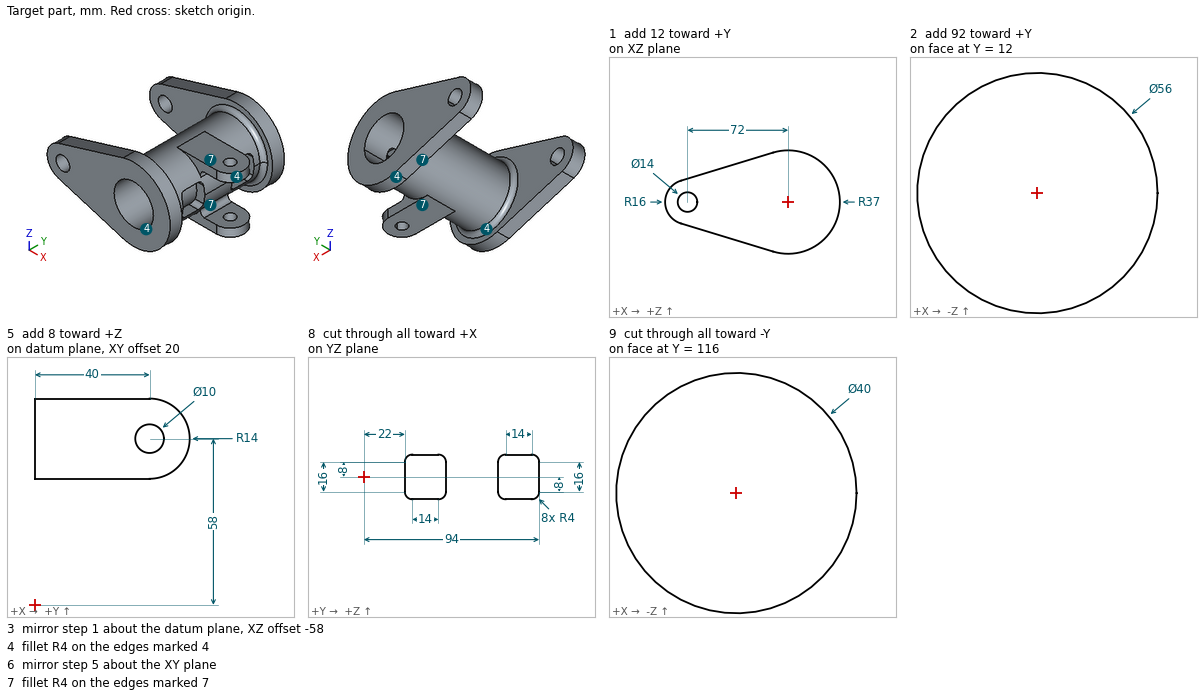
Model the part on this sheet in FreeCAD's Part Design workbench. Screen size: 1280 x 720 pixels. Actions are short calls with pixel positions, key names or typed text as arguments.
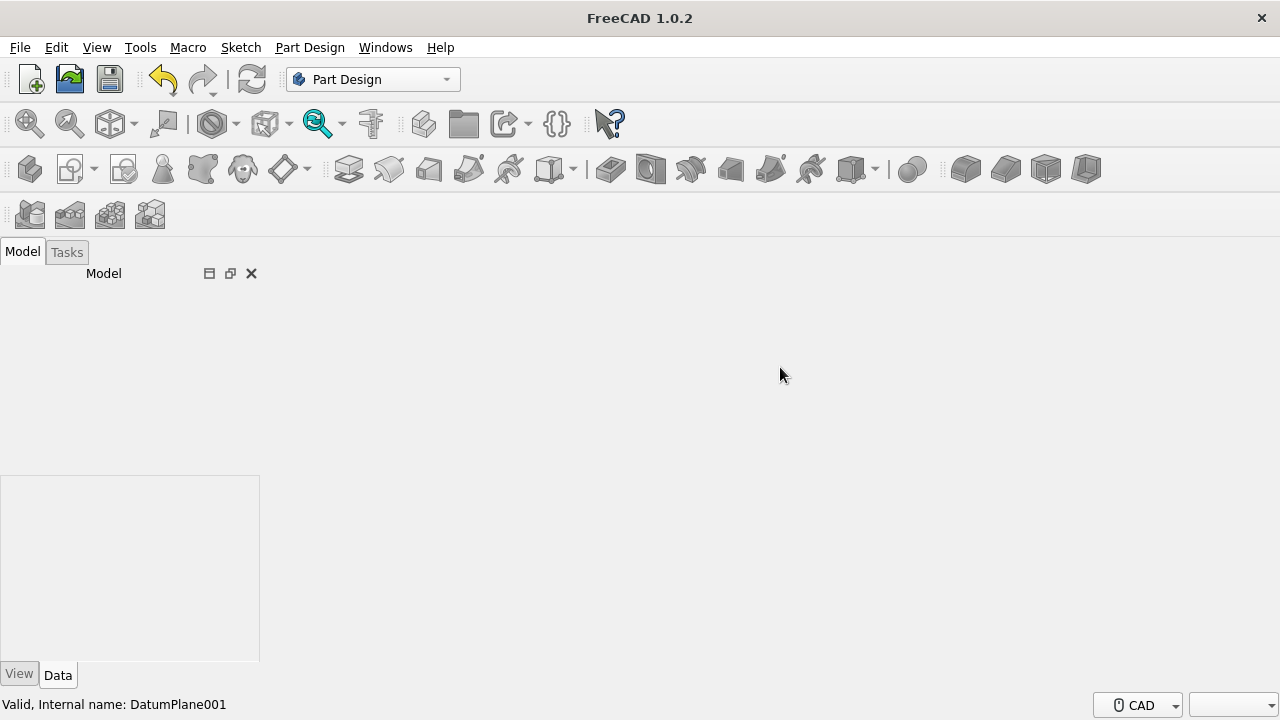
click(30, 80)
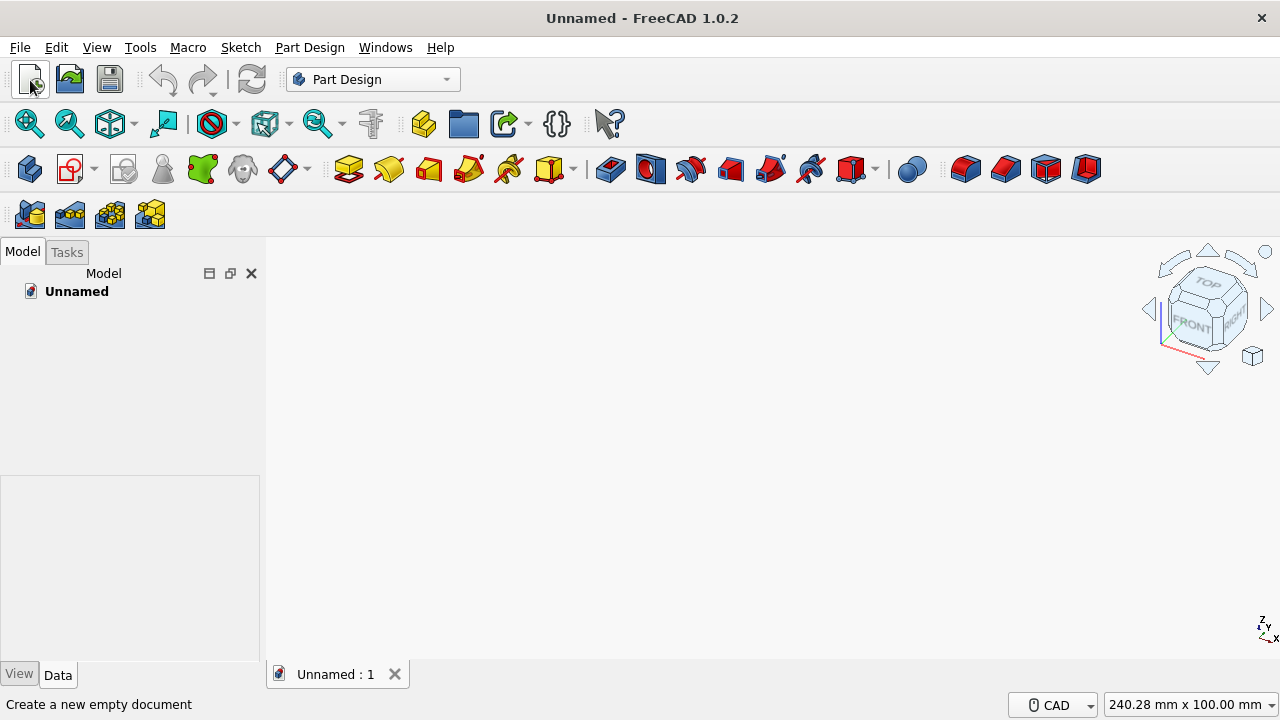
click(70, 170)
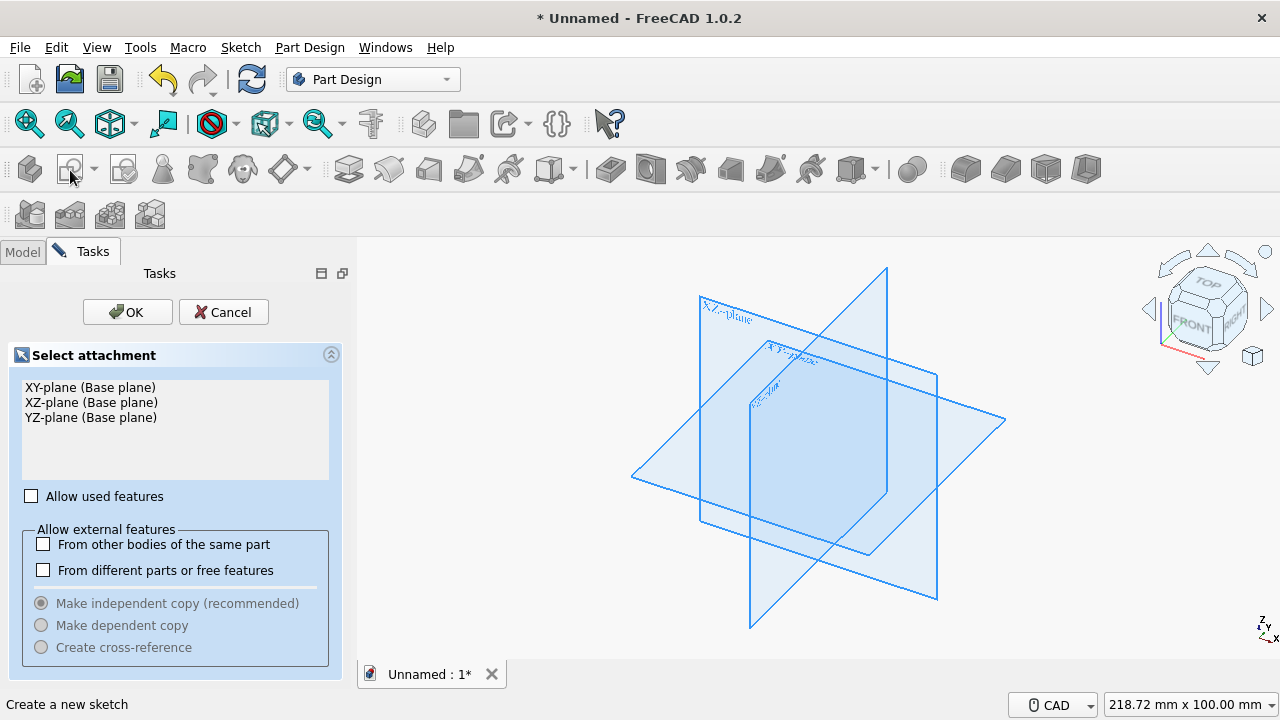
click(82, 402)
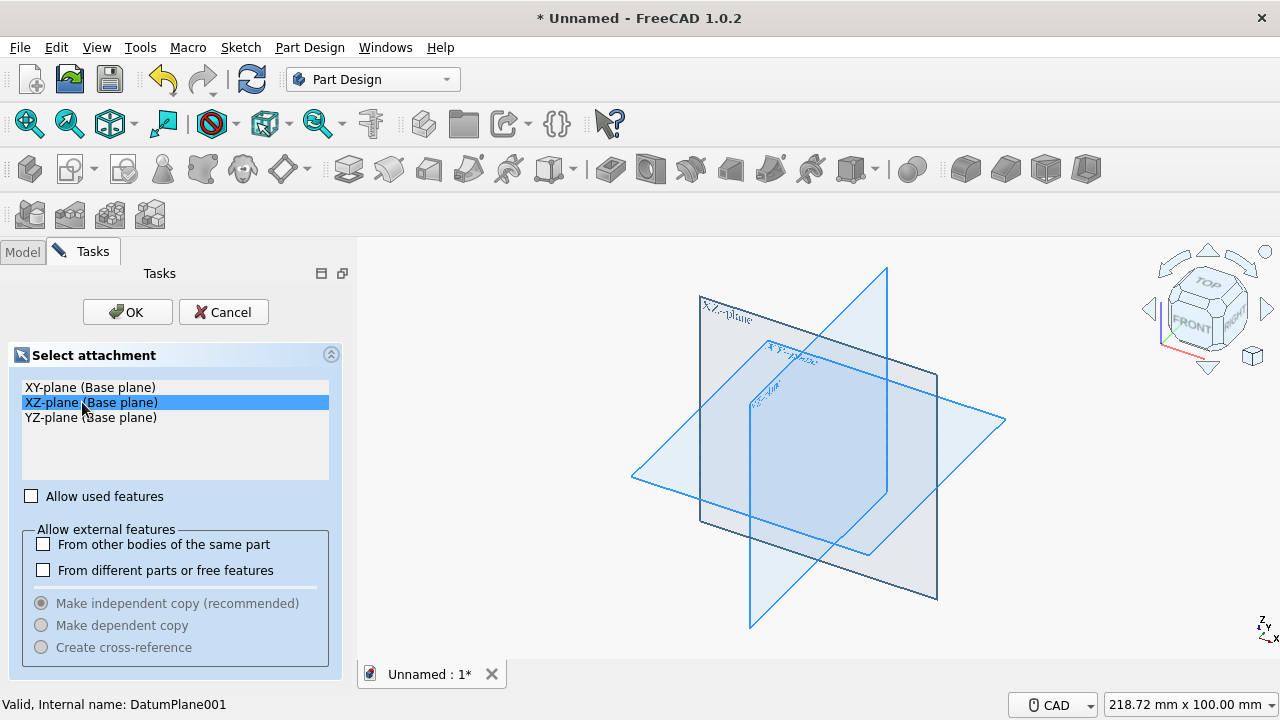
click(128, 312)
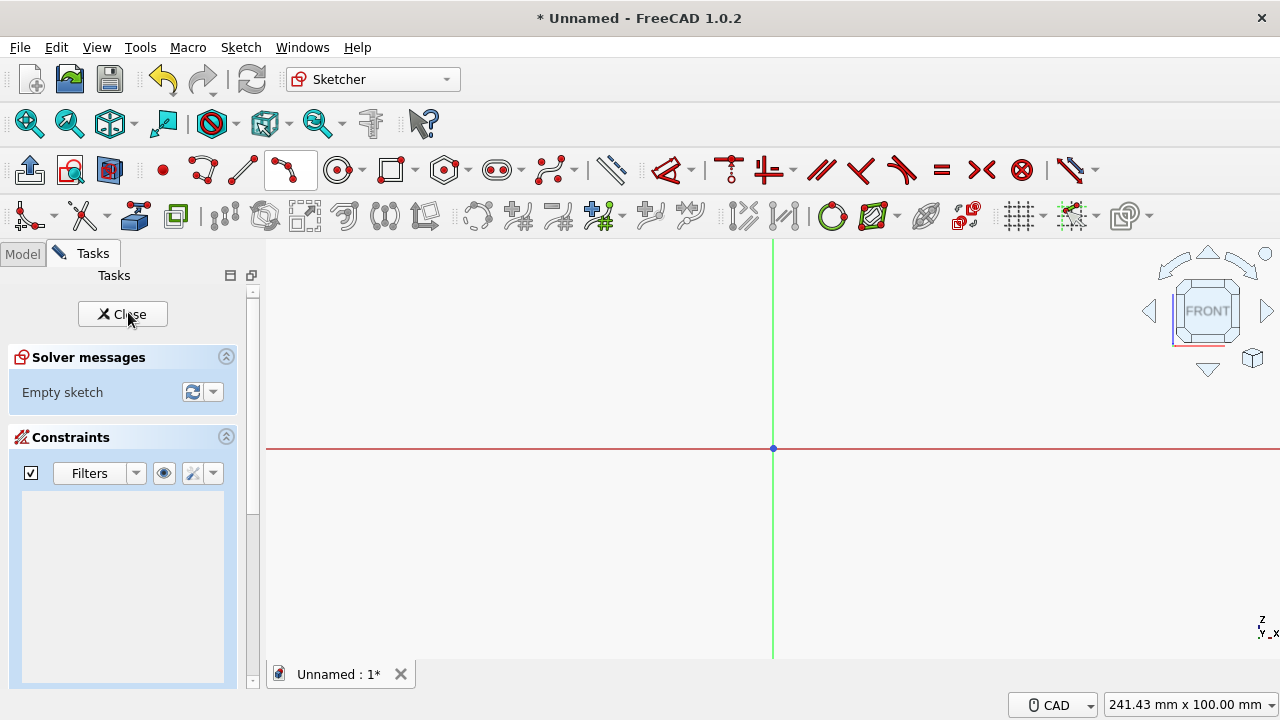
click(244, 170)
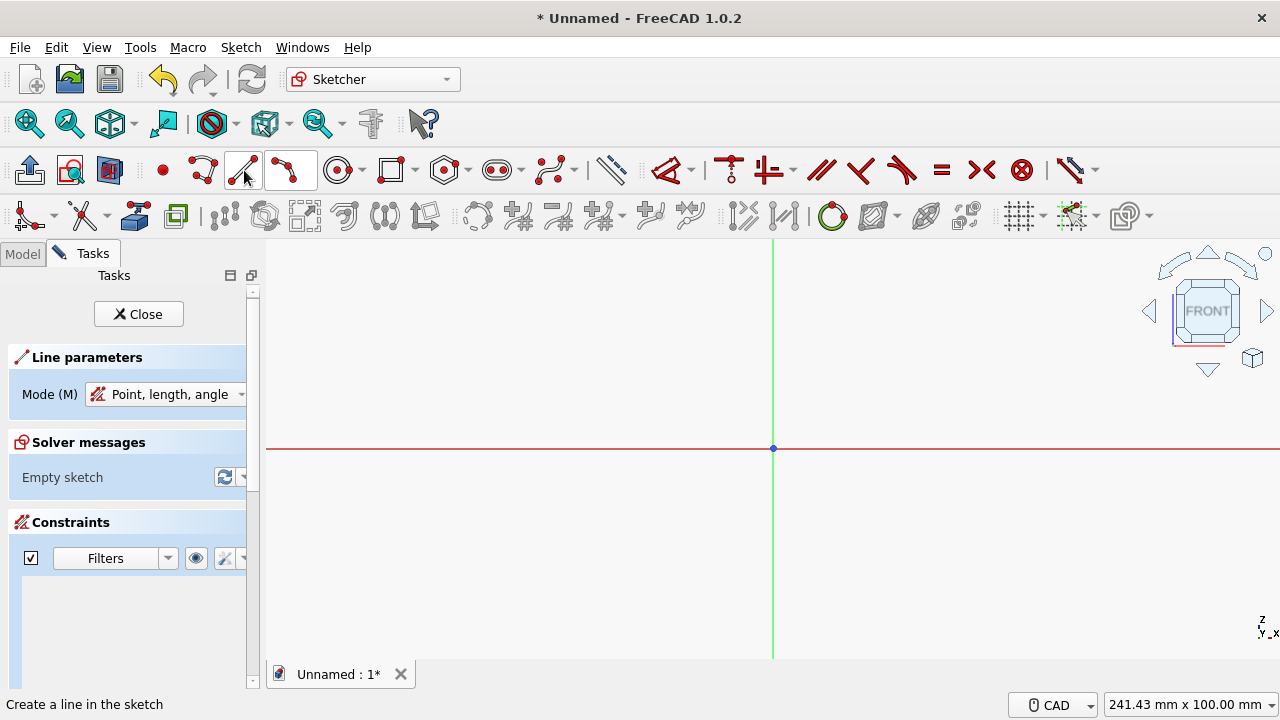
click(728, 598)
click(451, 513)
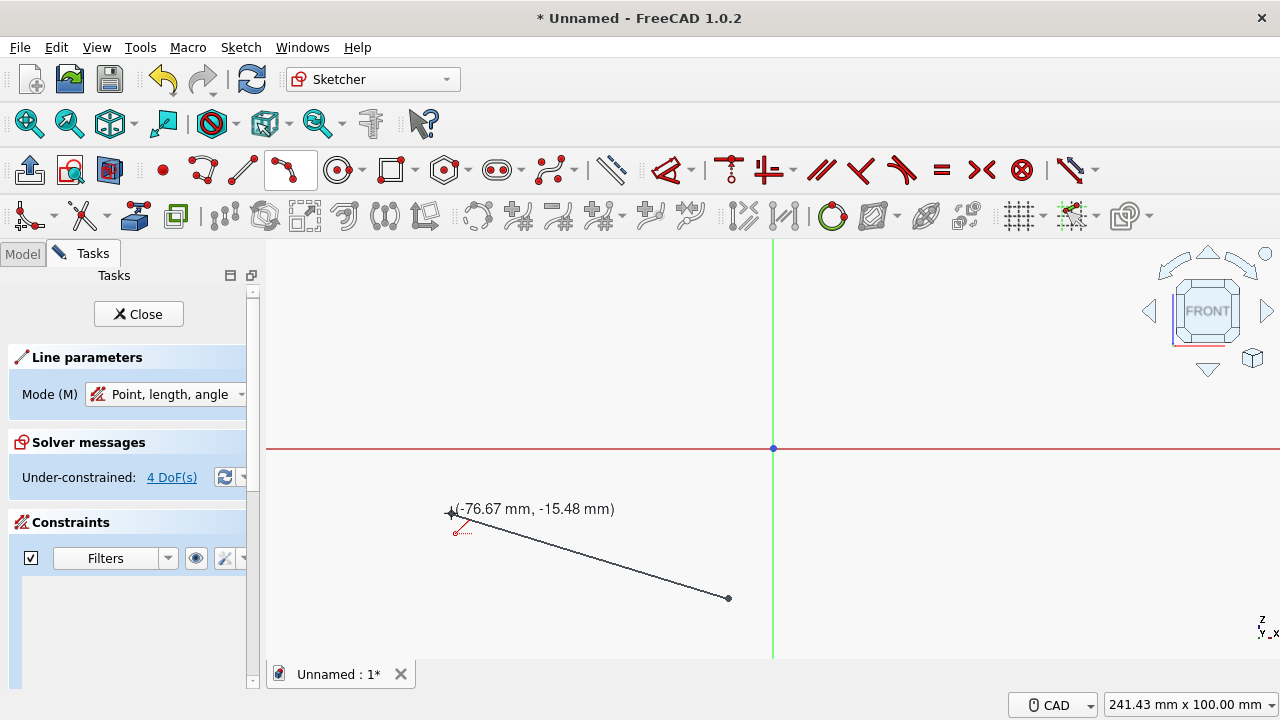
click(451, 385)
click(728, 300)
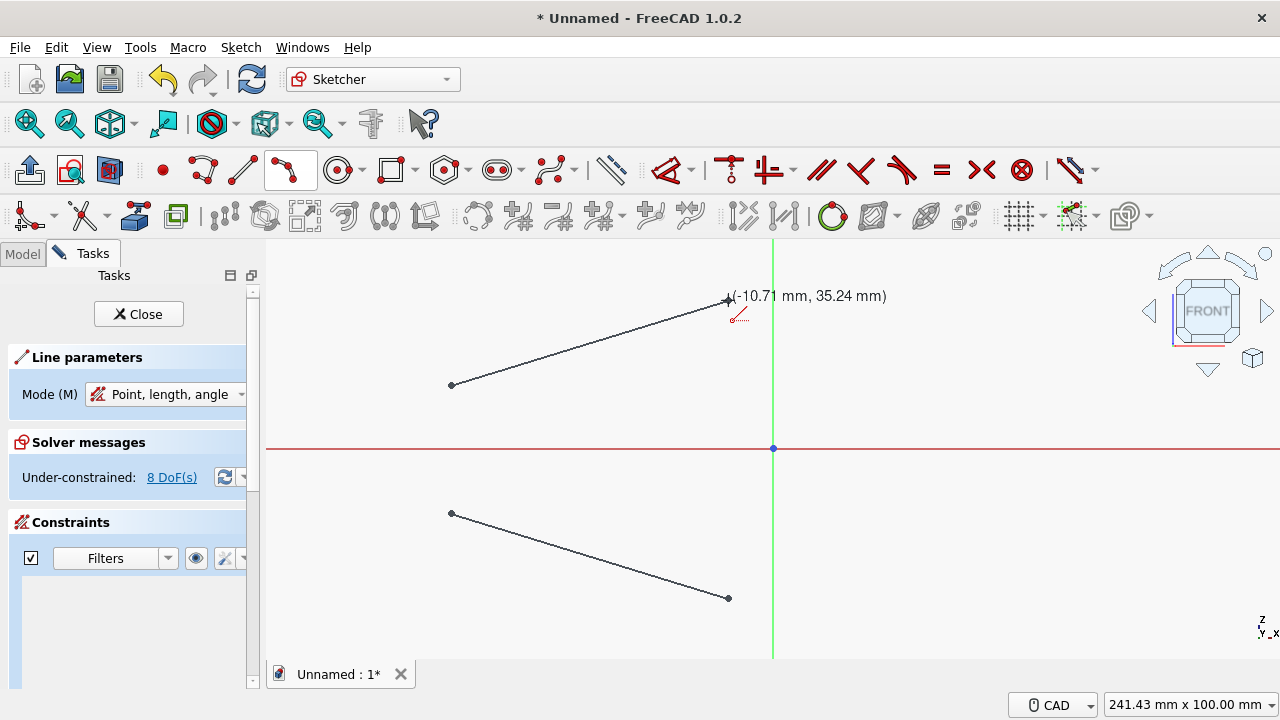
click(284, 170)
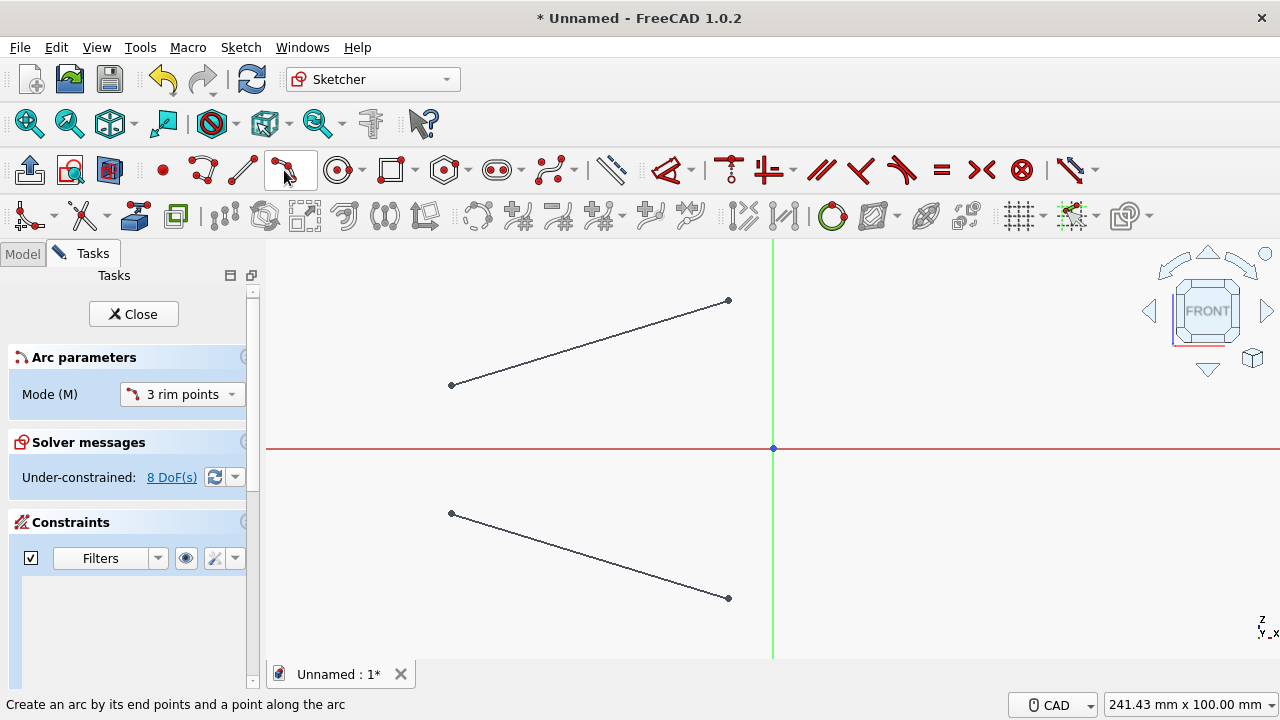
click(451, 514)
click(451, 386)
click(406, 432)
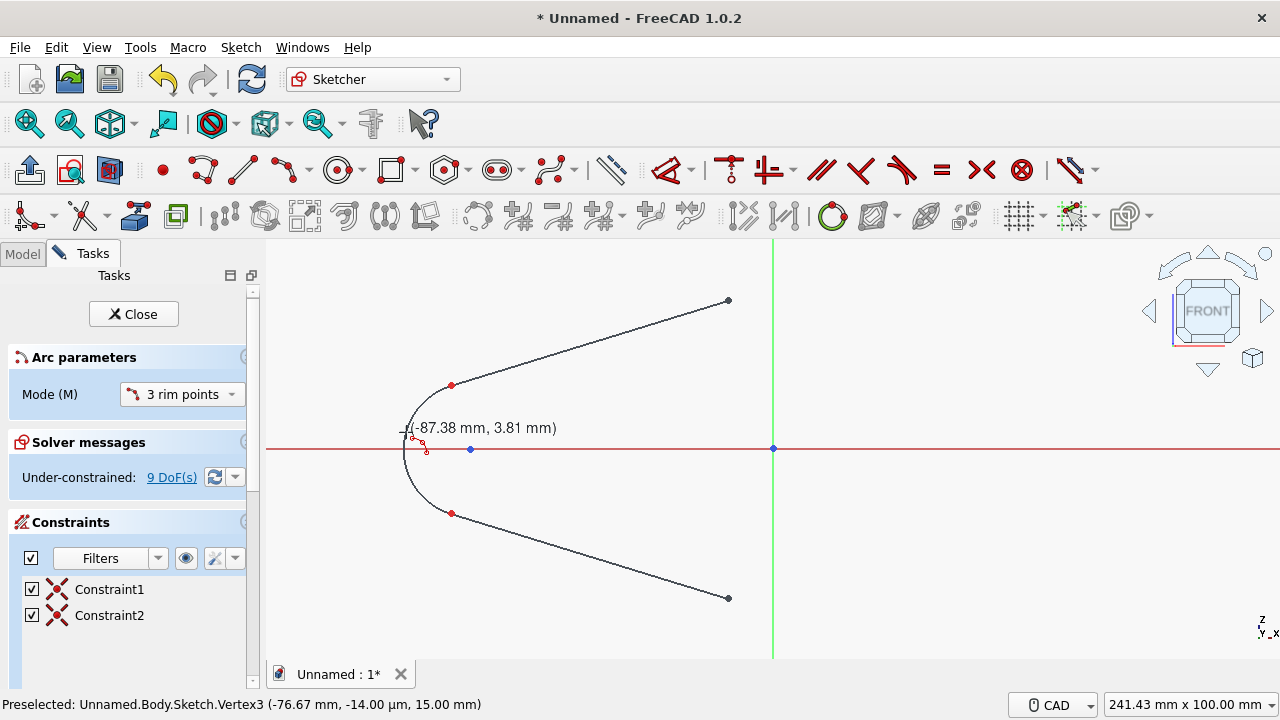
click(728, 301)
click(728, 599)
click(918, 506)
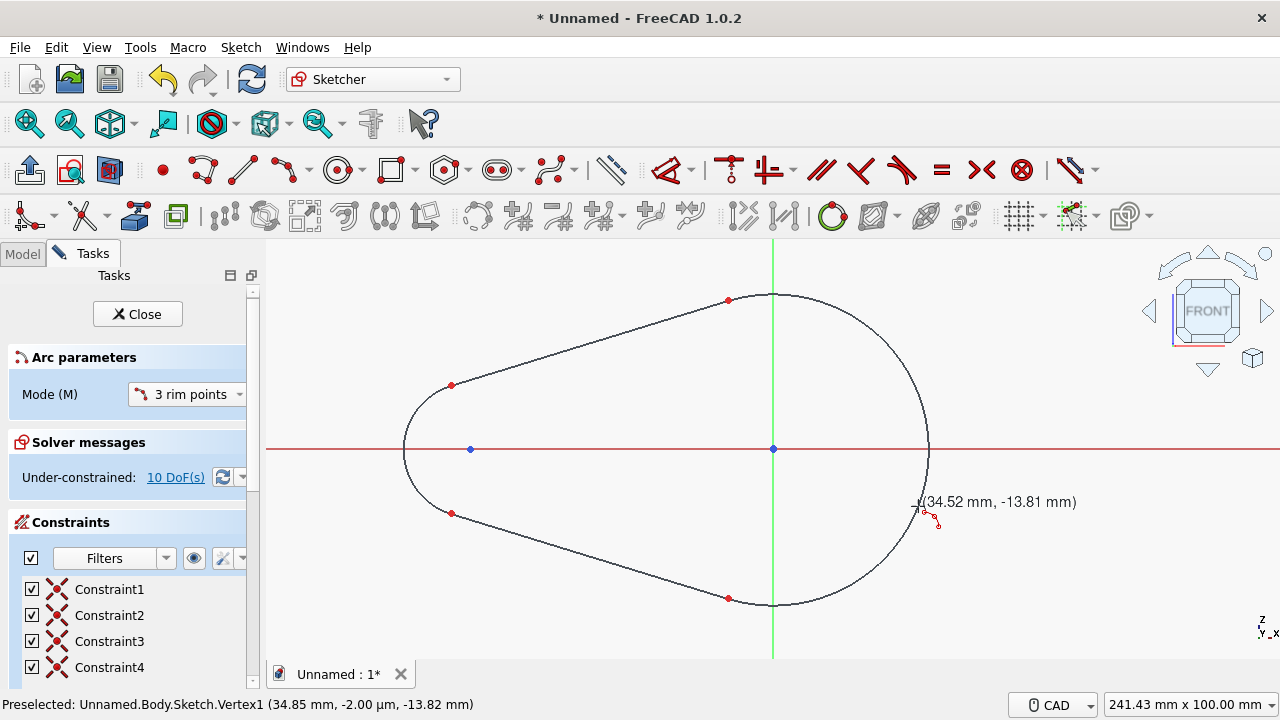
click(338, 170)